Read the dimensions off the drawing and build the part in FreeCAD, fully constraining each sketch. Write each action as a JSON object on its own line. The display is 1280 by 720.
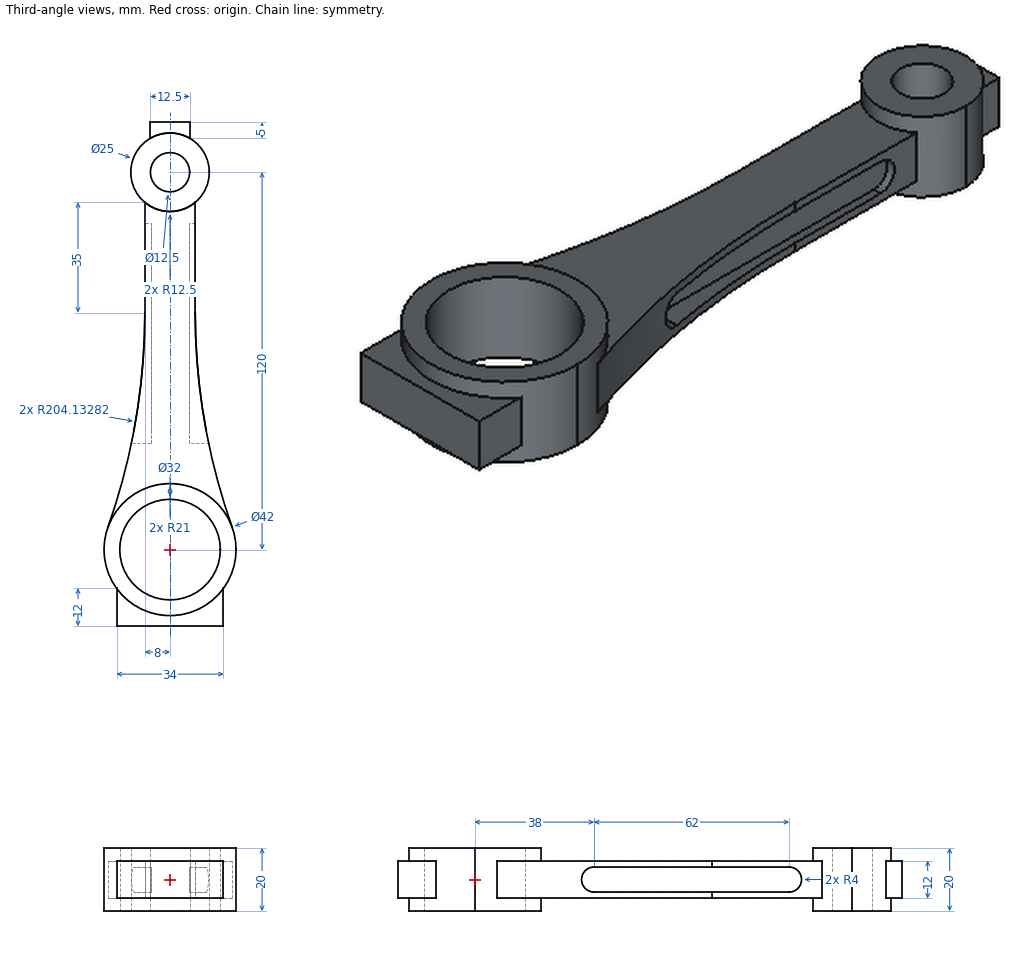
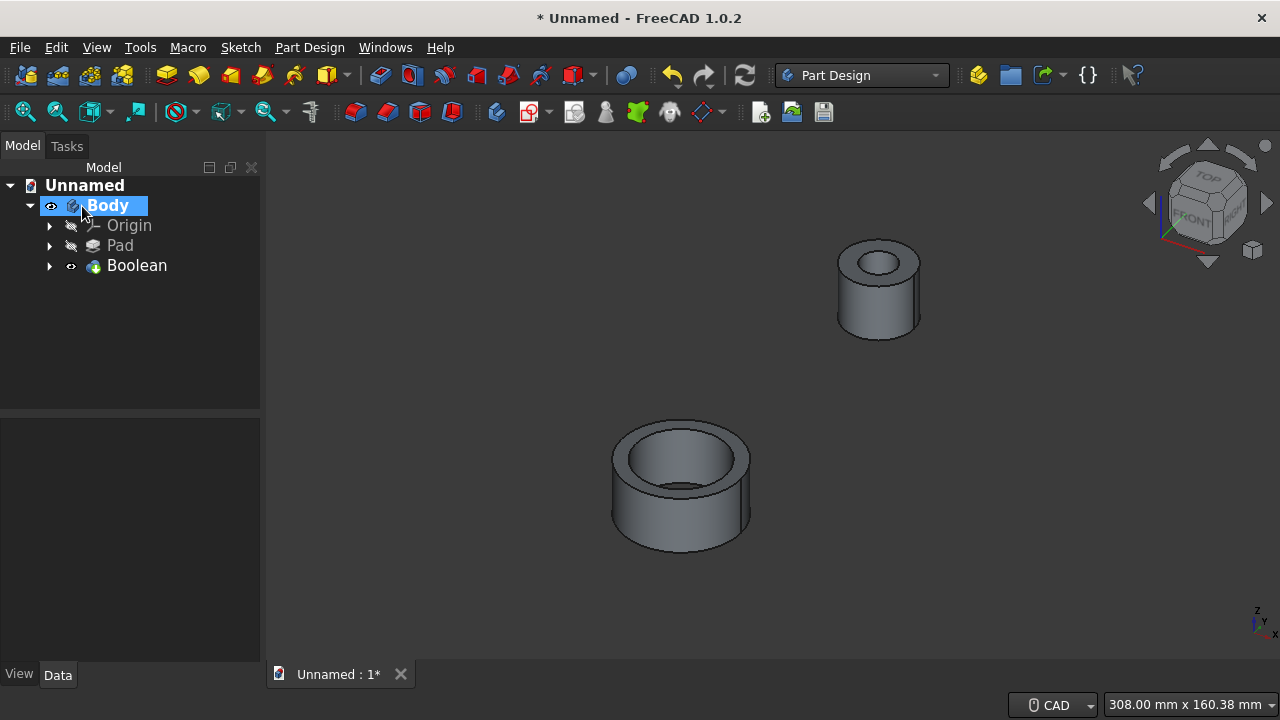
{"action": "left_click", "coordinate": [530, 112]}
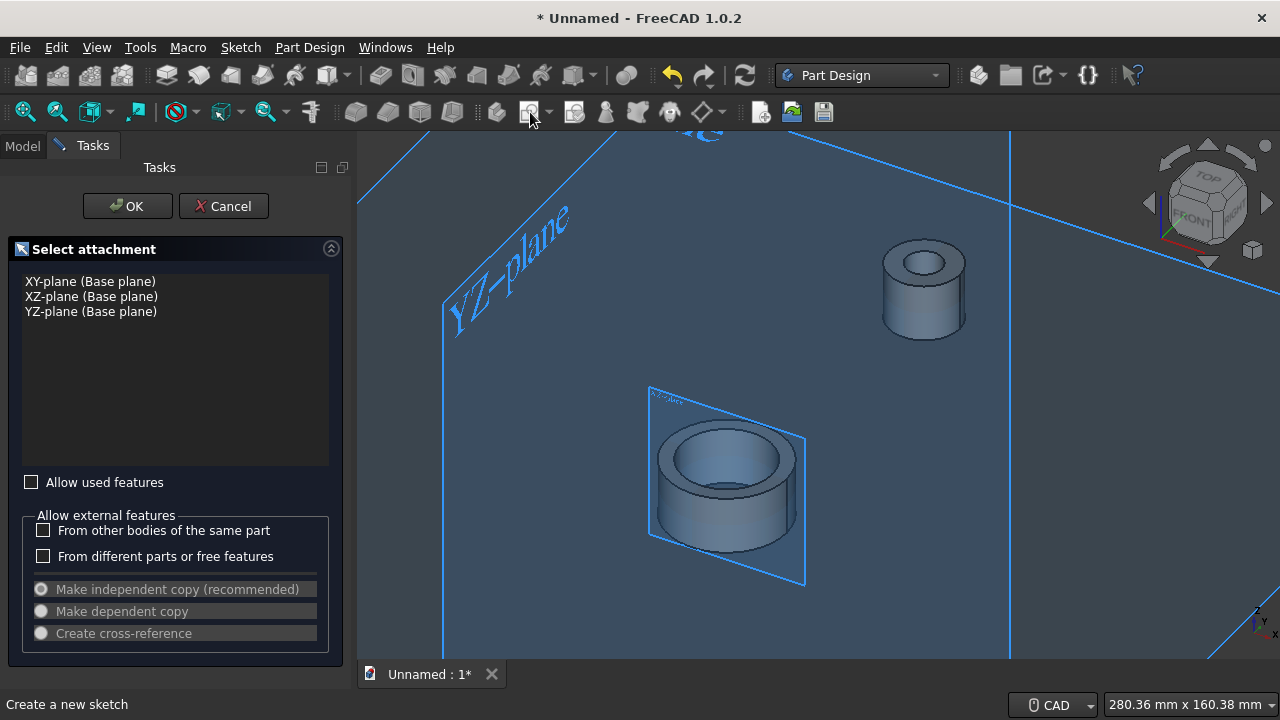
{"action": "left_click", "coordinate": [82, 282]}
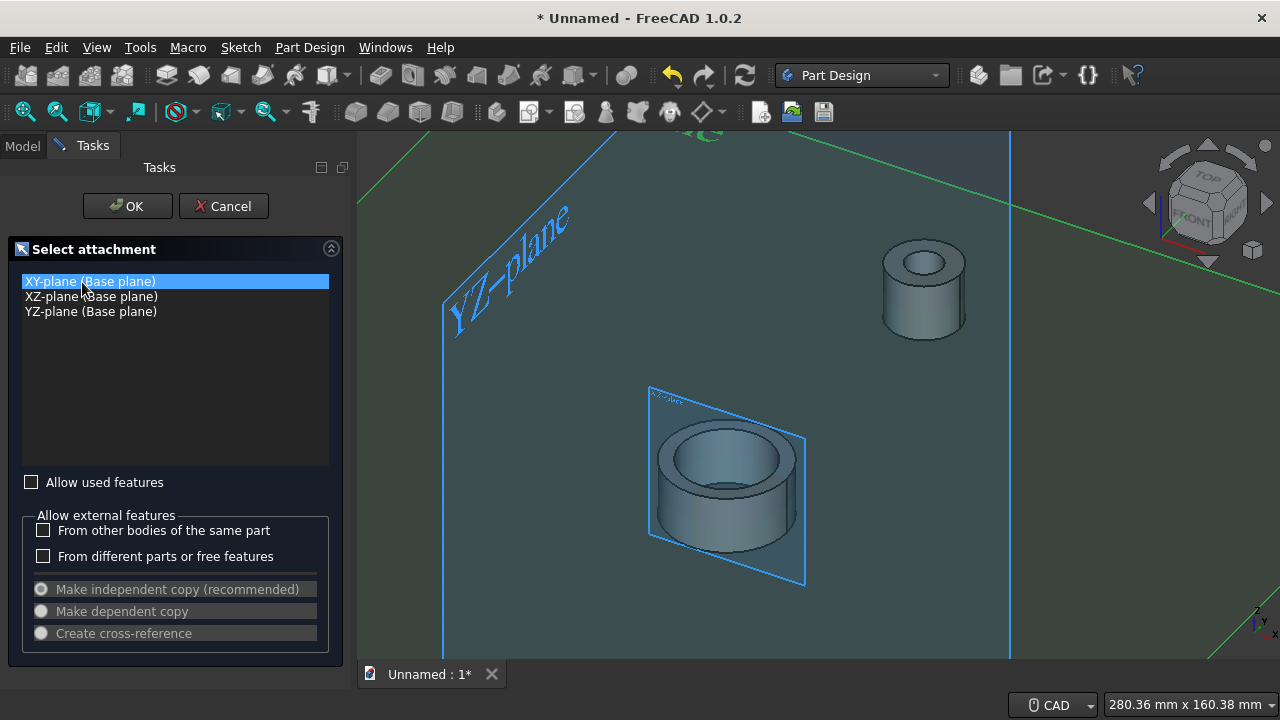
{"action": "left_click", "coordinate": [128, 206]}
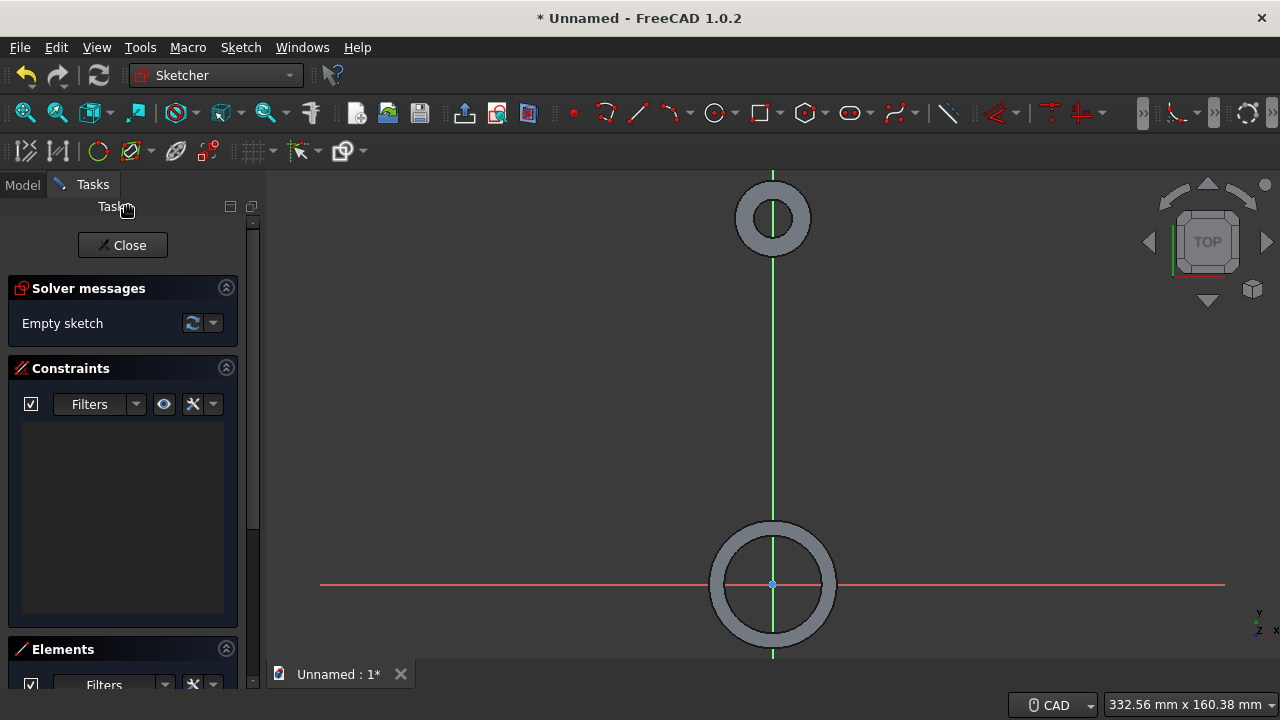
{"action": "left_click", "coordinate": [530, 114]}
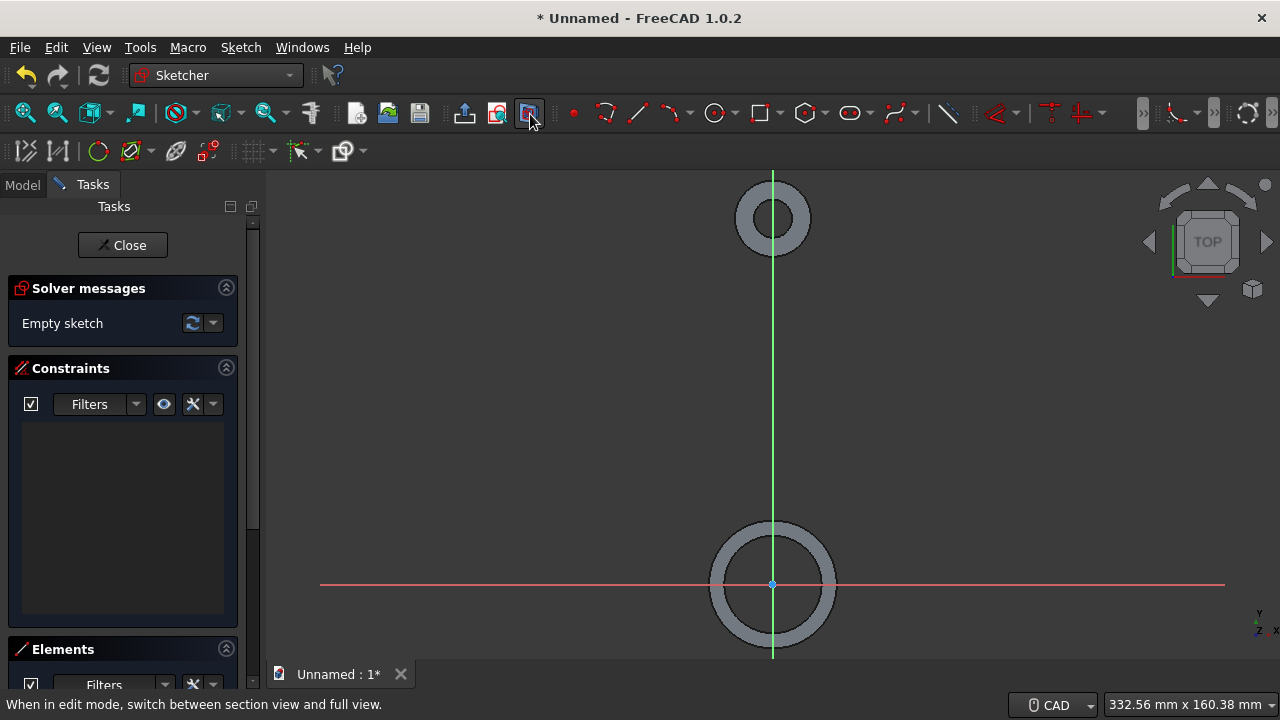
{"action": "scroll", "coordinate": [565, 414], "scroll_direction": "down", "scroll_amount": 2}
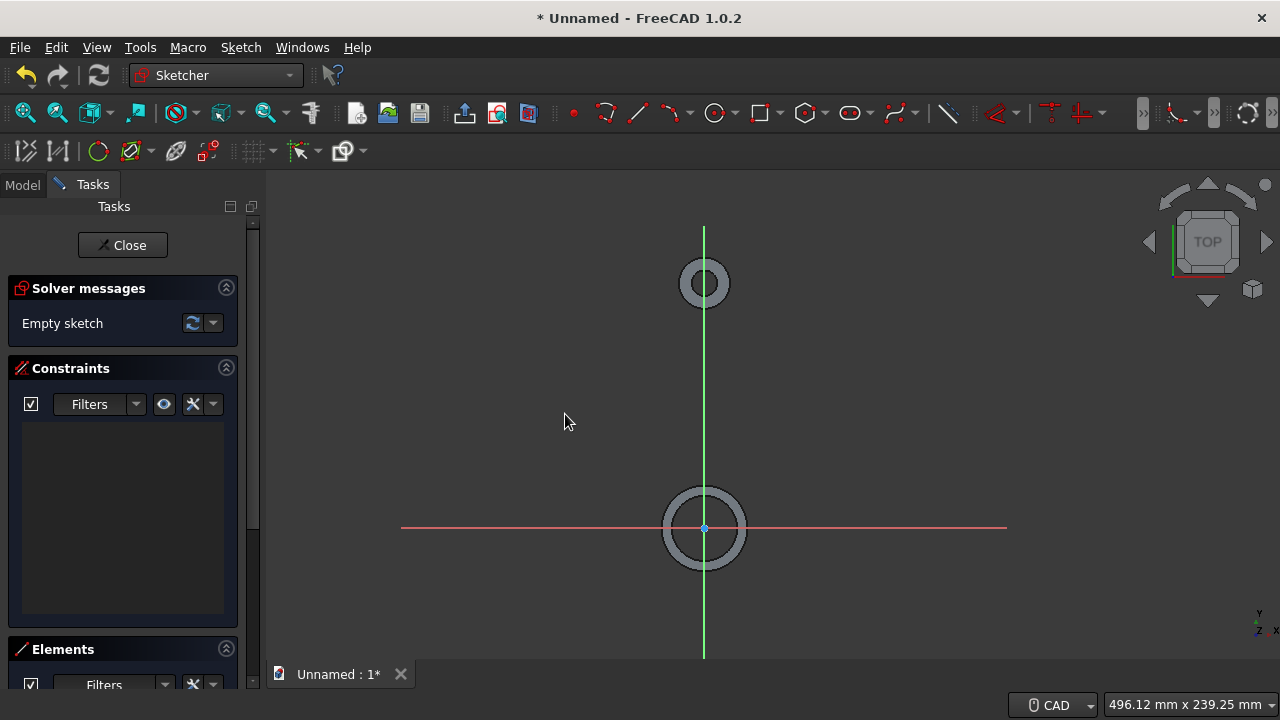
{"action": "key", "text": "g l"}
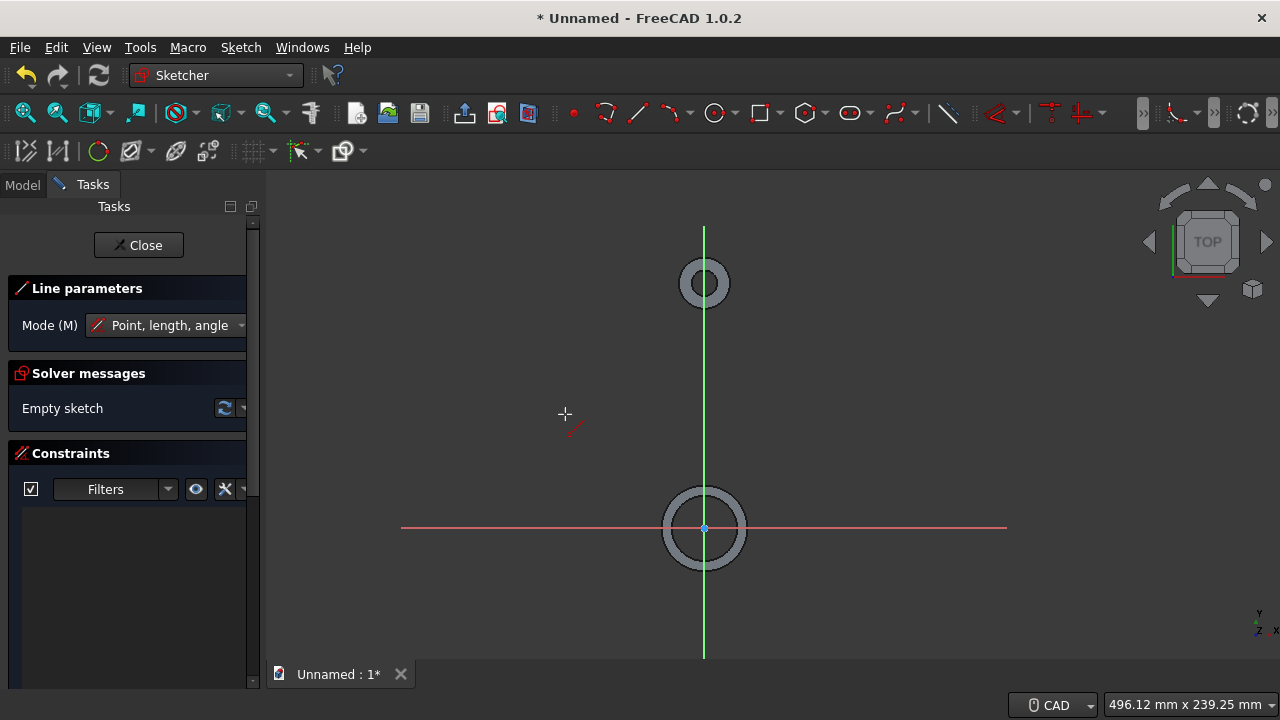
{"action": "left_click", "coordinate": [688, 303]}
{"action": "left_click", "coordinate": [688, 374]}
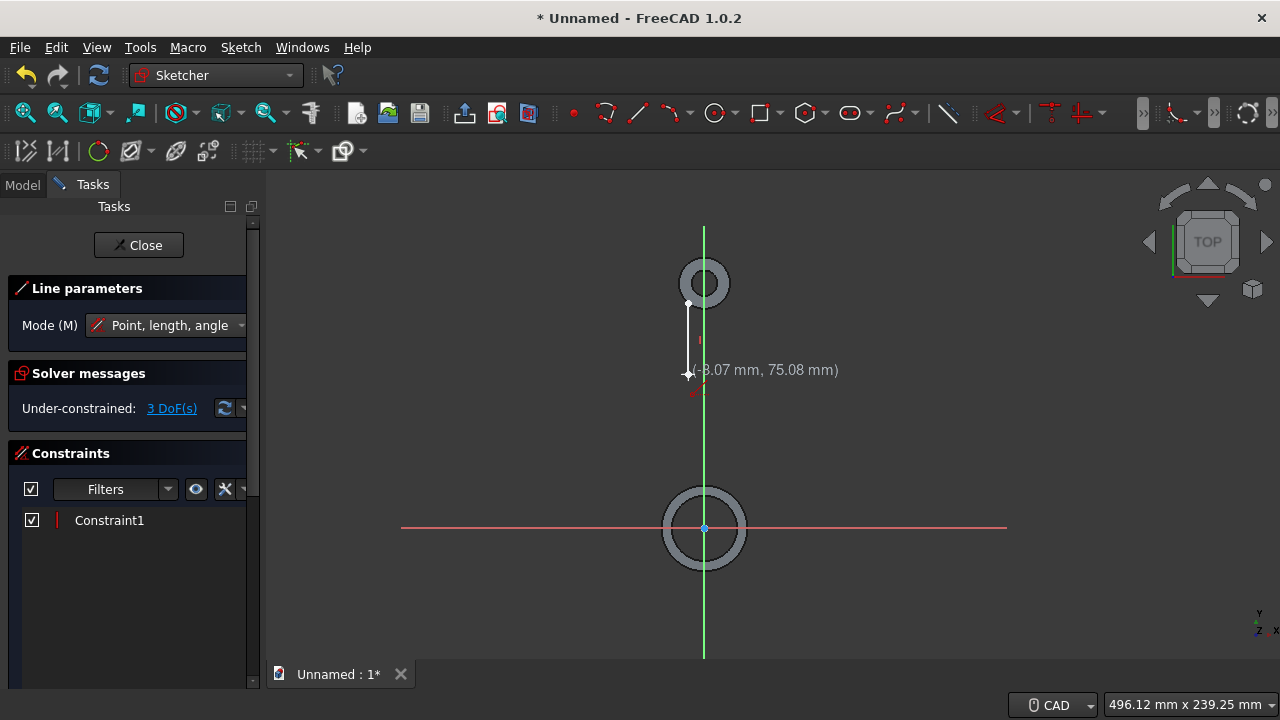
{"action": "left_click", "coordinate": [721, 374]}
{"action": "left_click", "coordinate": [721, 303]}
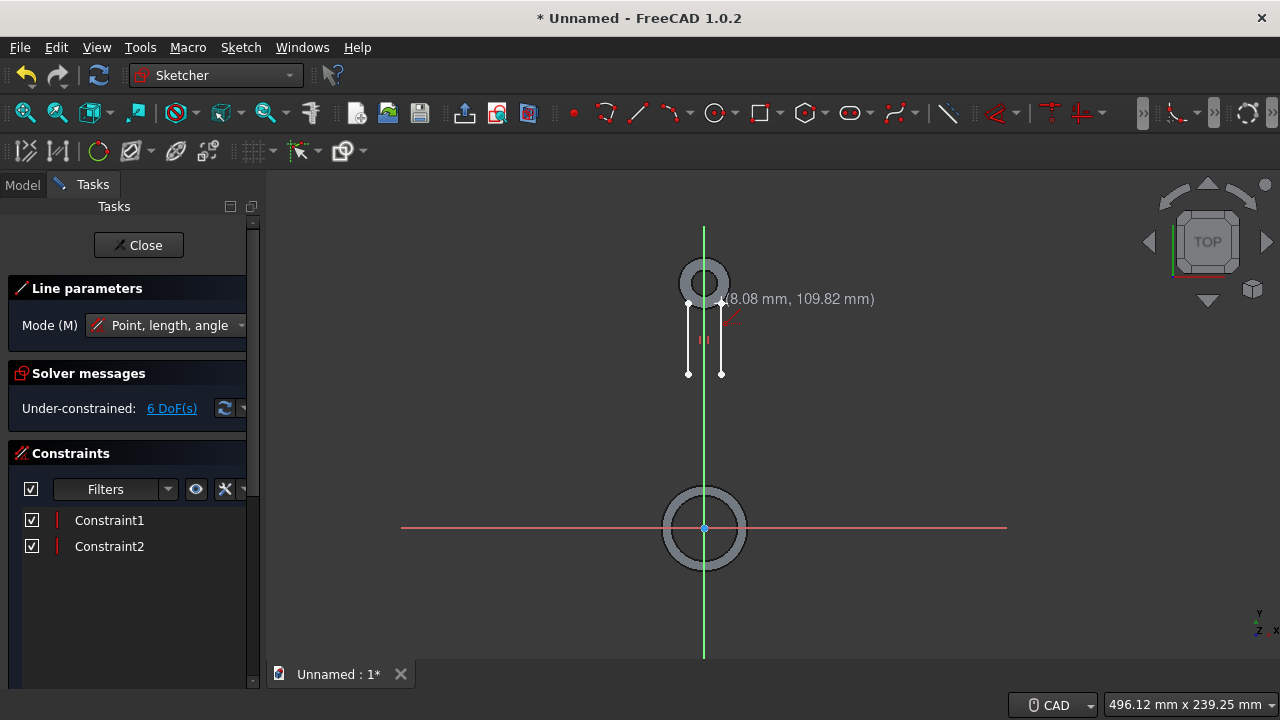
{"action": "key", "text": "g 3 a"}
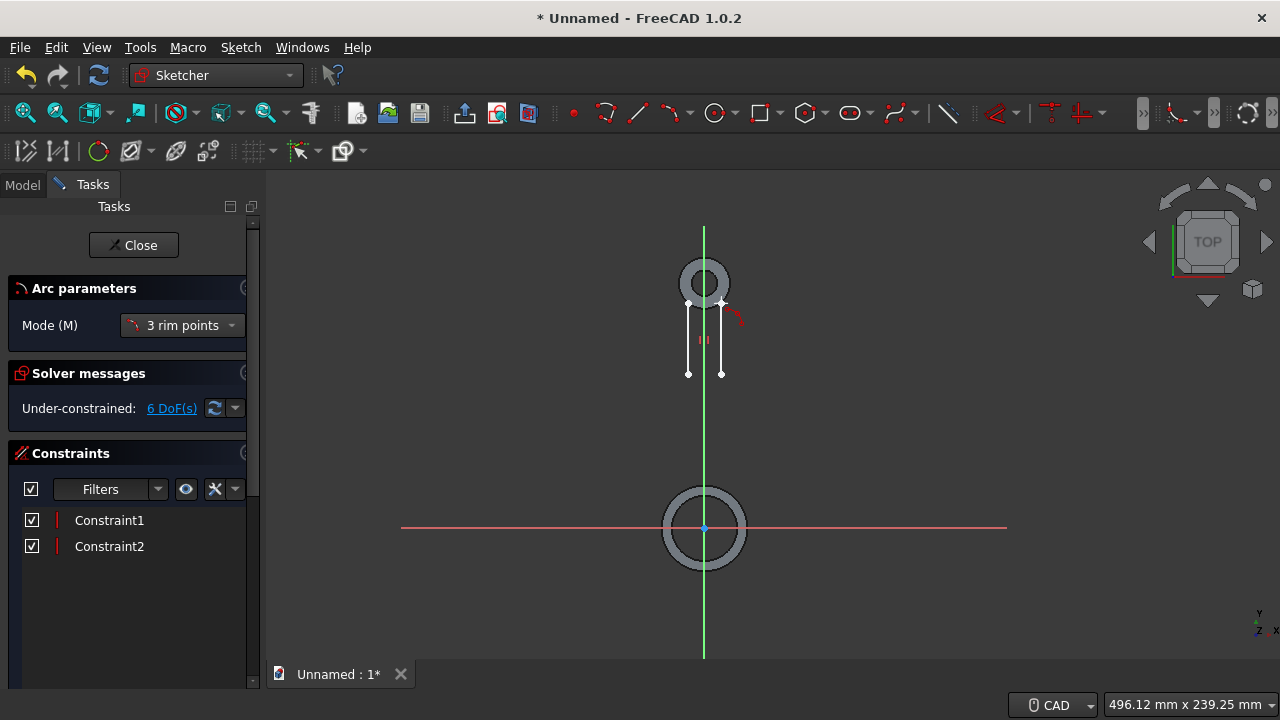
{"action": "left_click", "coordinate": [688, 375]}
{"action": "left_click", "coordinate": [664, 514]}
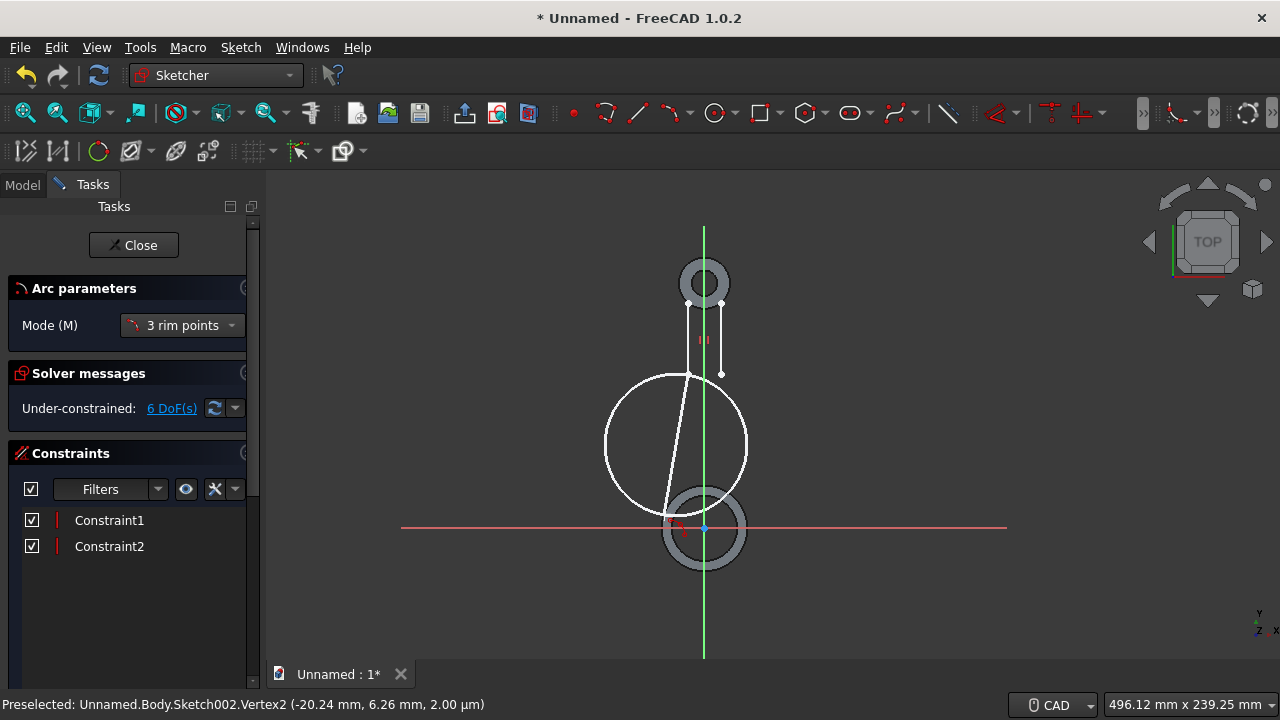
{"action": "scroll", "coordinate": [682, 445], "scroll_direction": "up", "scroll_amount": 5}